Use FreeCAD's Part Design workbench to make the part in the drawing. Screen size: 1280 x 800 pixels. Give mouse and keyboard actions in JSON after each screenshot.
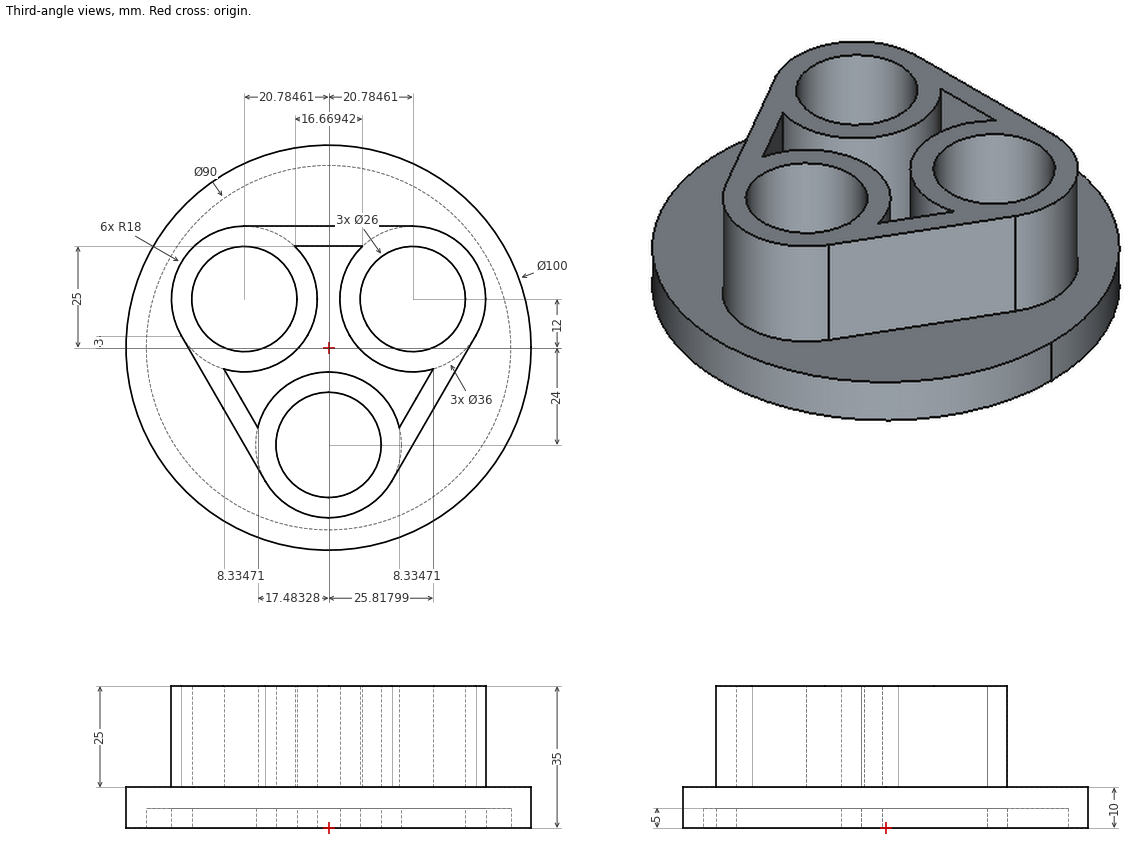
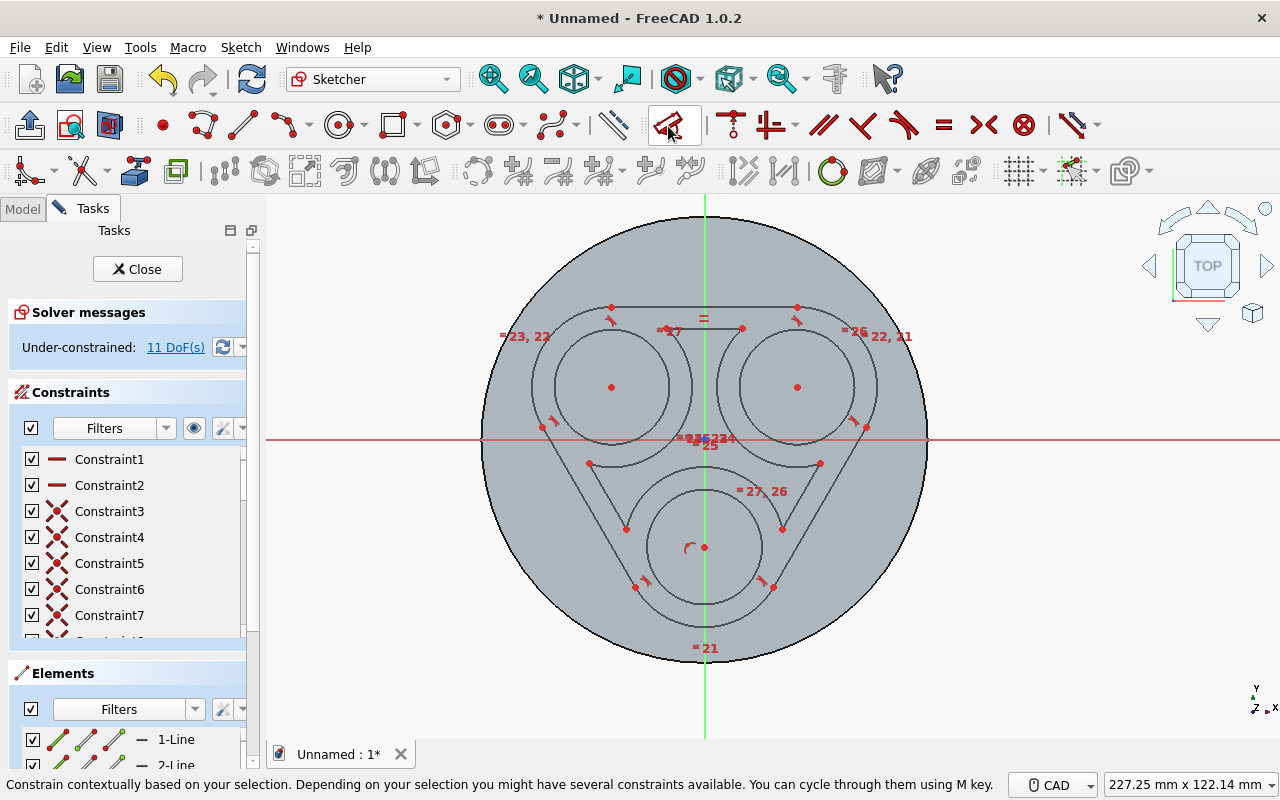
{"action": "left_click", "coordinate": [672, 620]}
{"action": "left_click", "coordinate": [659, 649]}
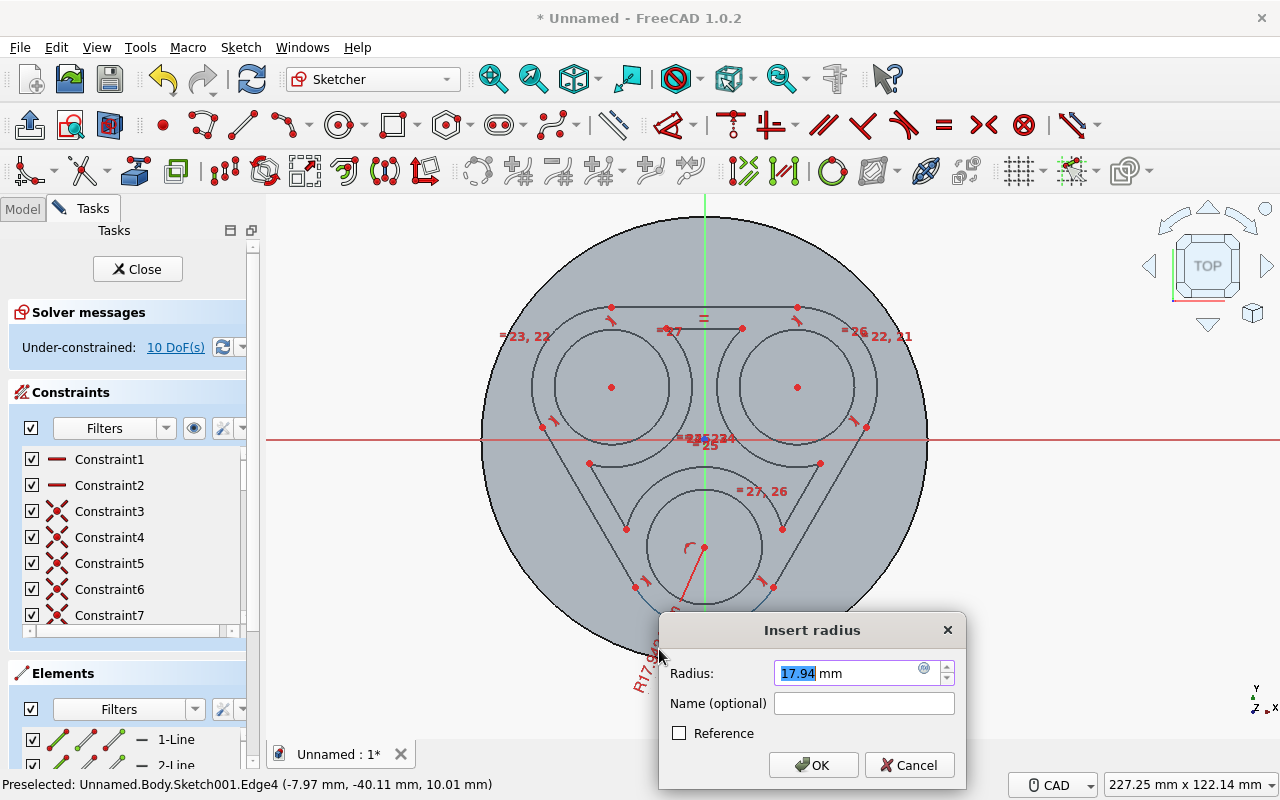
{"action": "type", "text": "18"}
{"action": "key", "text": "Return"}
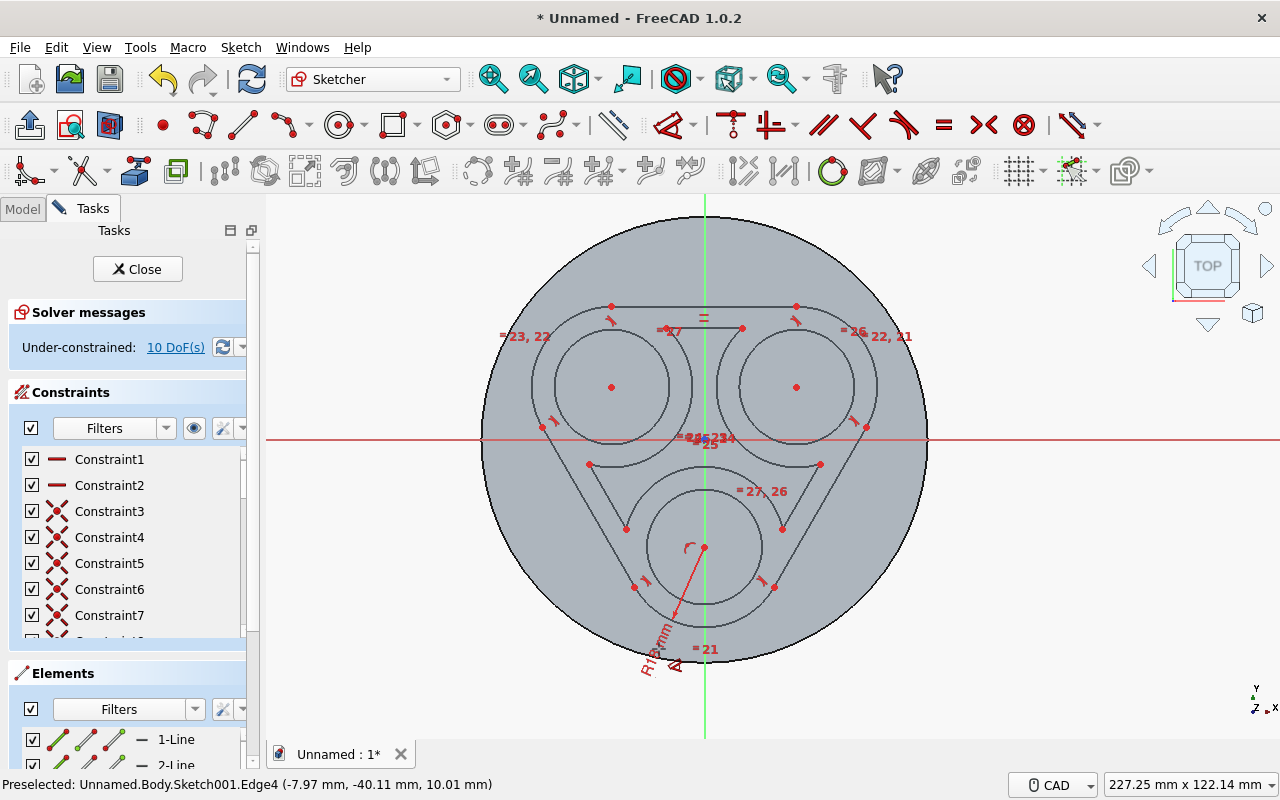
{"action": "left_click", "coordinate": [837, 346]}
{"action": "left_click", "coordinate": [875, 307]}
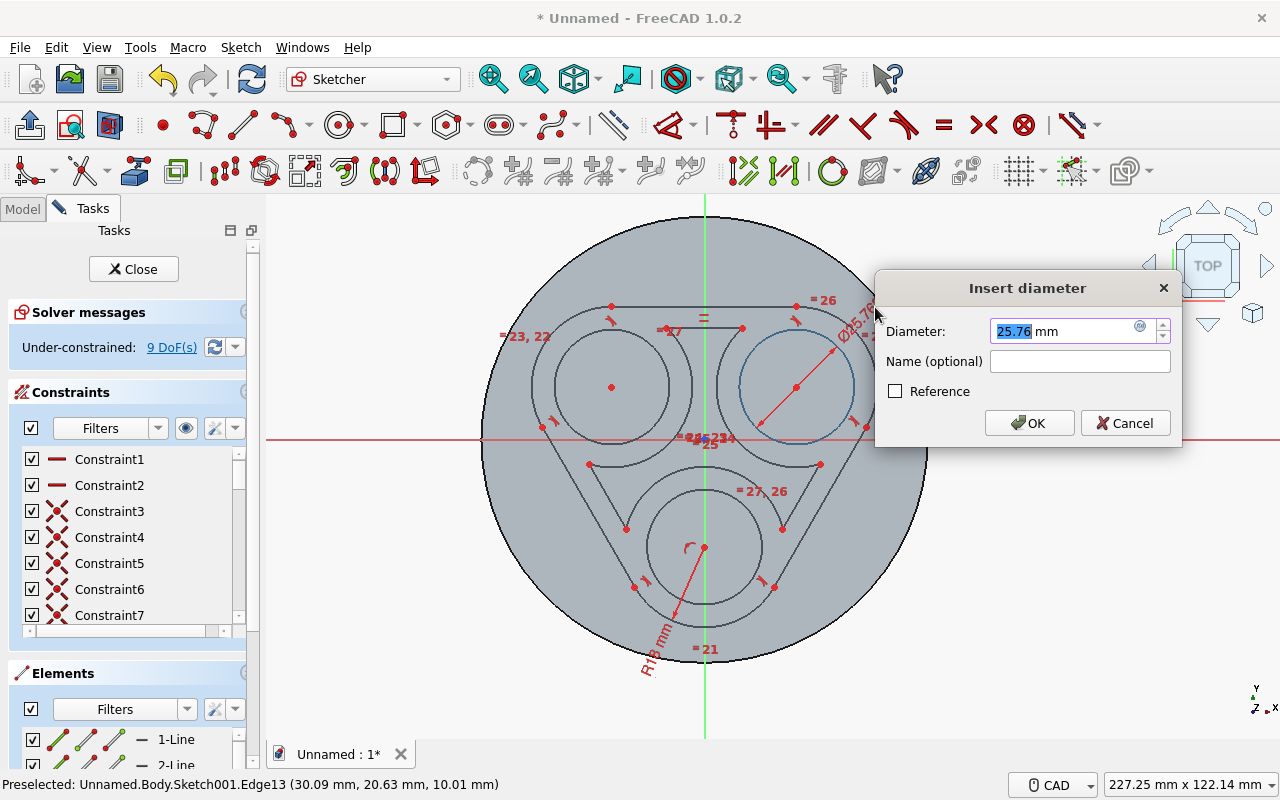
{"action": "type", "text": "26"}
{"action": "key", "text": "Return"}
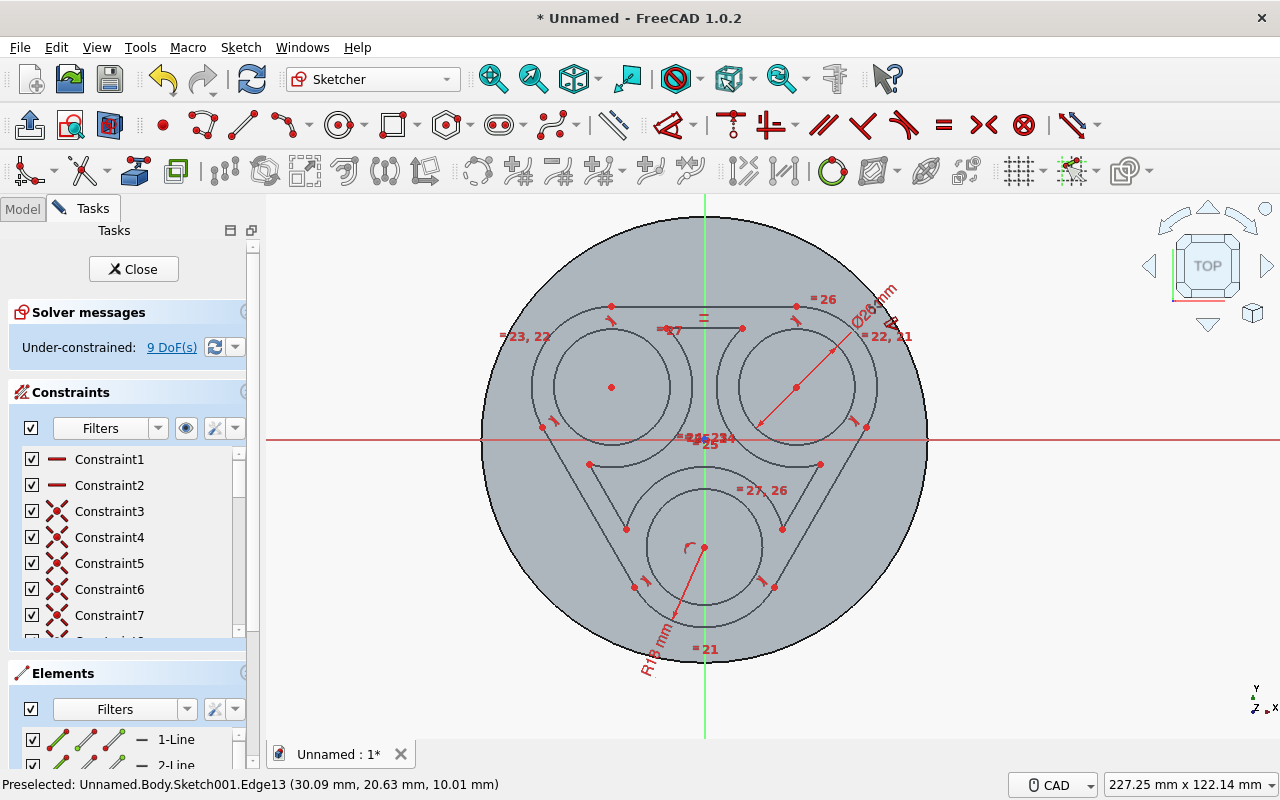
{"action": "scroll", "coordinate": [542, 427], "scroll_direction": "up", "scroll_amount": 6}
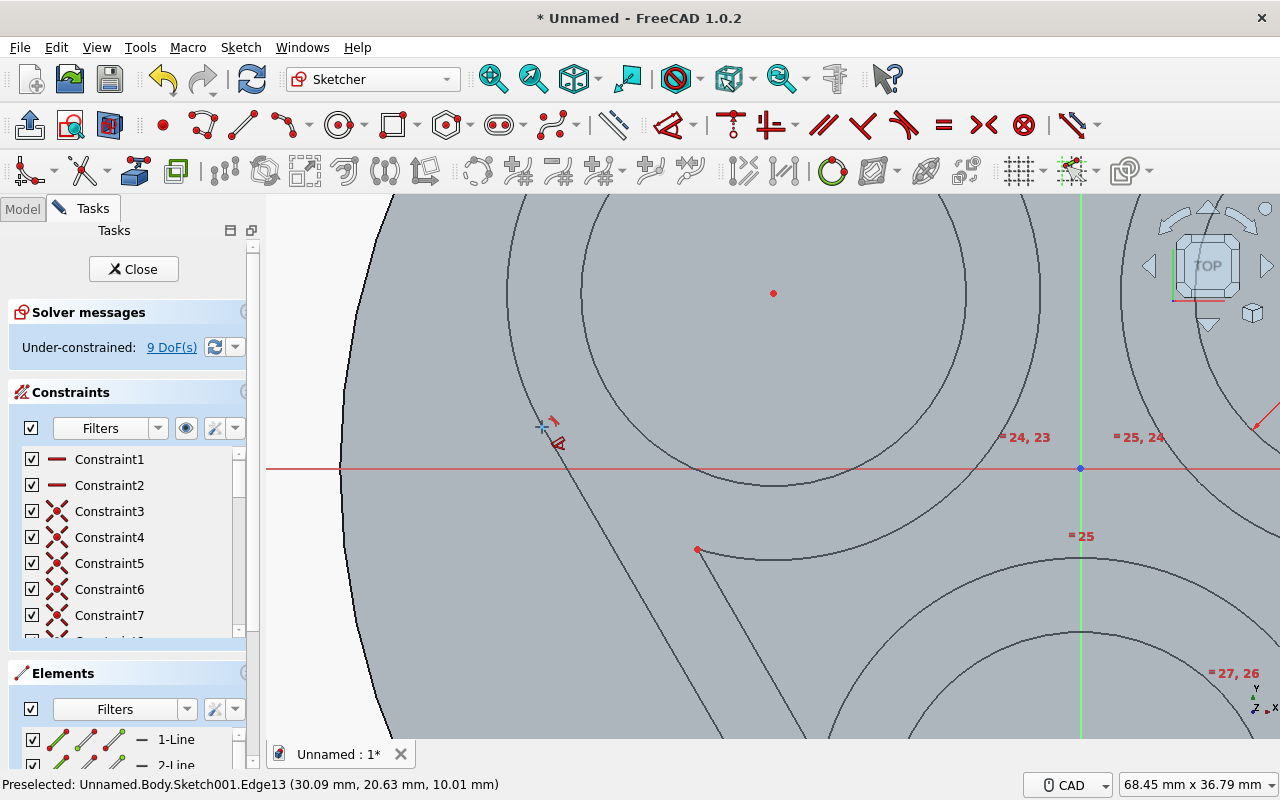
{"action": "left_click", "coordinate": [543, 427]}
{"action": "left_click", "coordinate": [509, 448]}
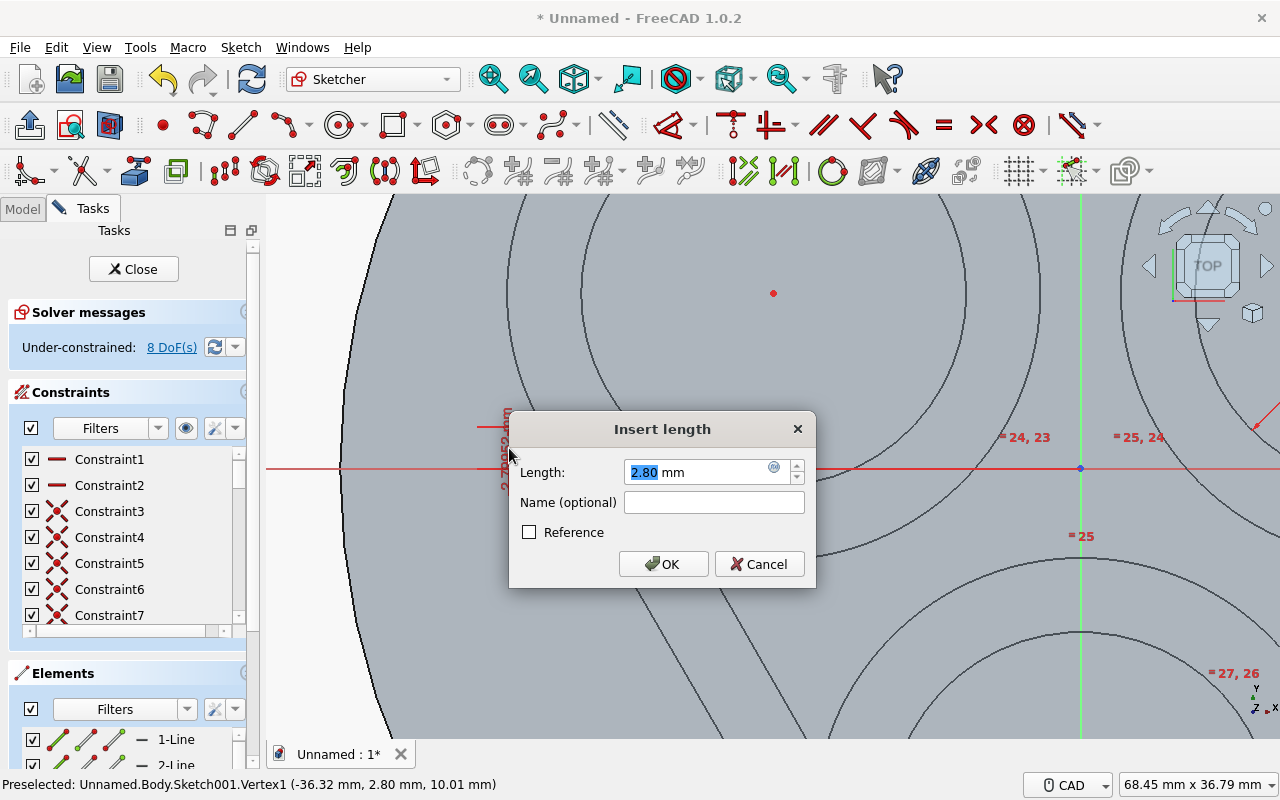
{"action": "type", "text": "3"}
{"action": "key", "text": "Return"}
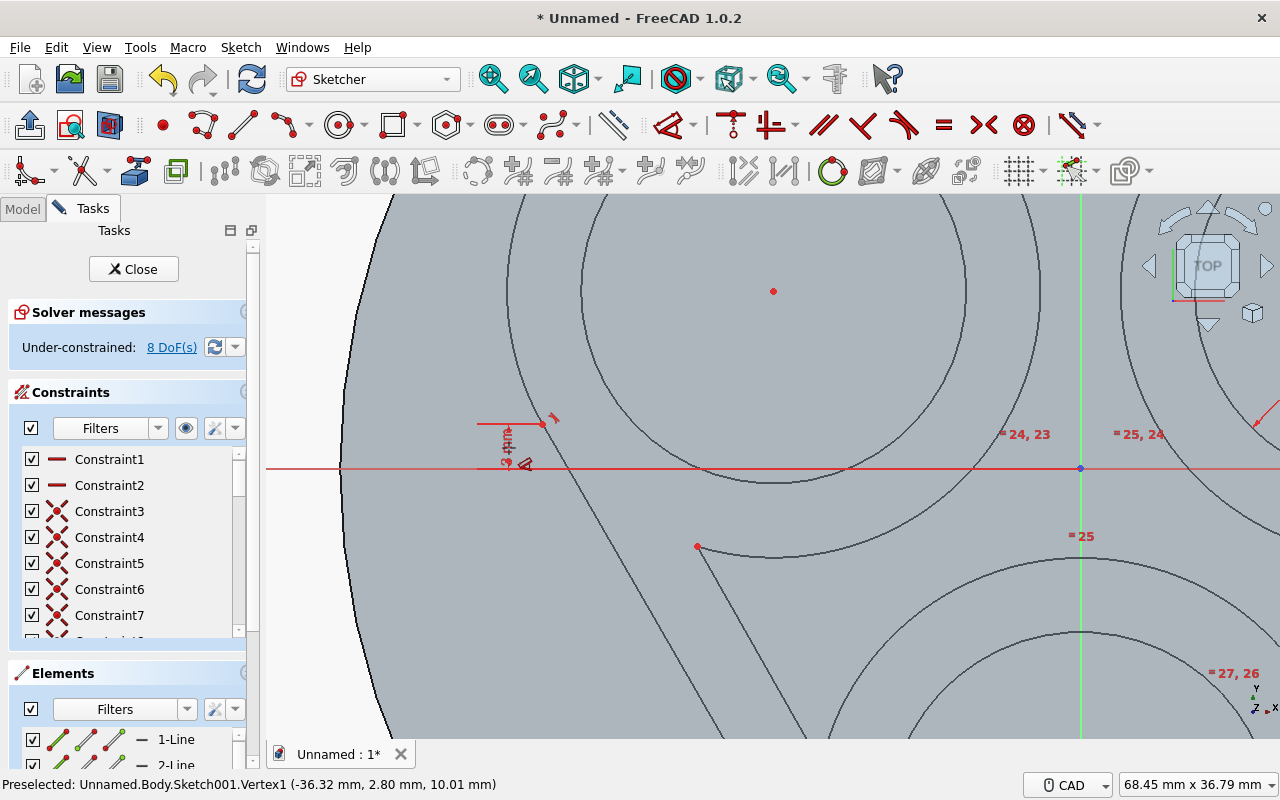
{"action": "scroll", "coordinate": [542, 427], "scroll_direction": "down", "scroll_amount": 6}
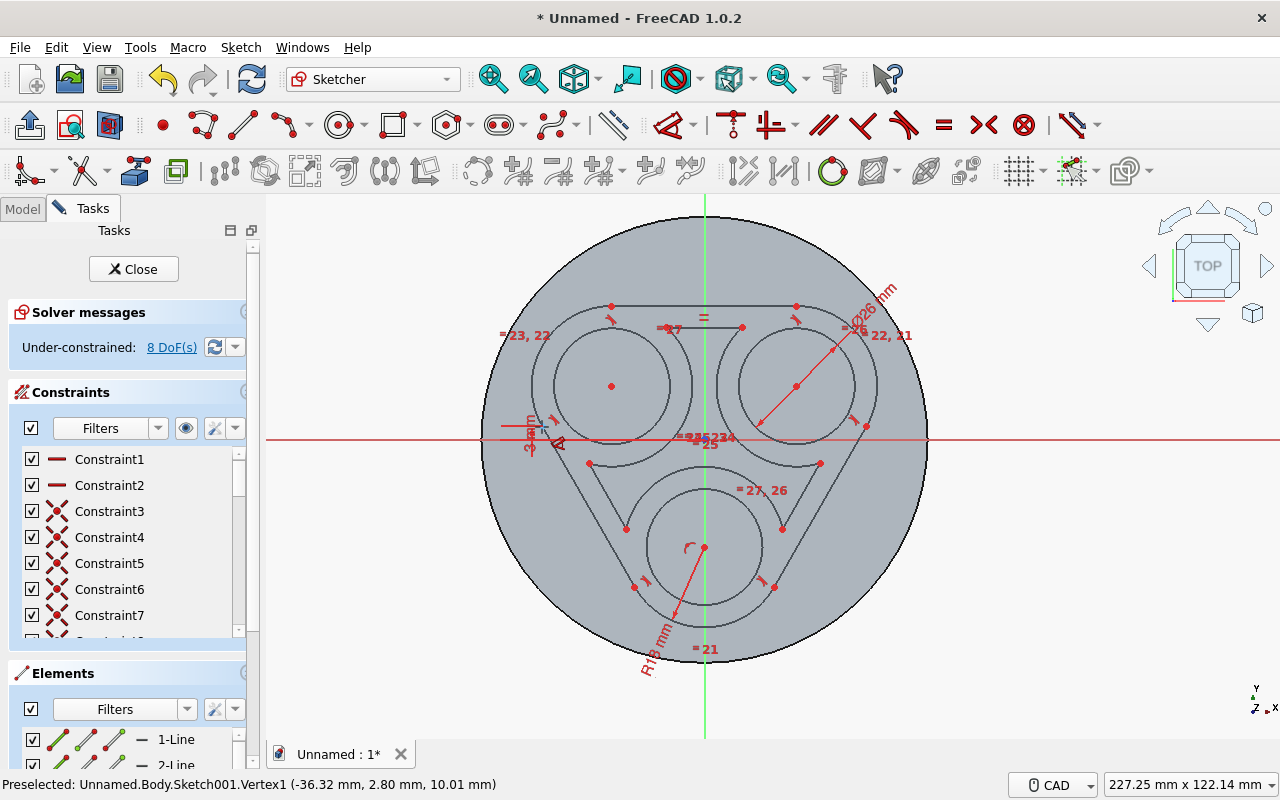
{"action": "scroll", "coordinate": [866, 426], "scroll_direction": "up", "scroll_amount": 6}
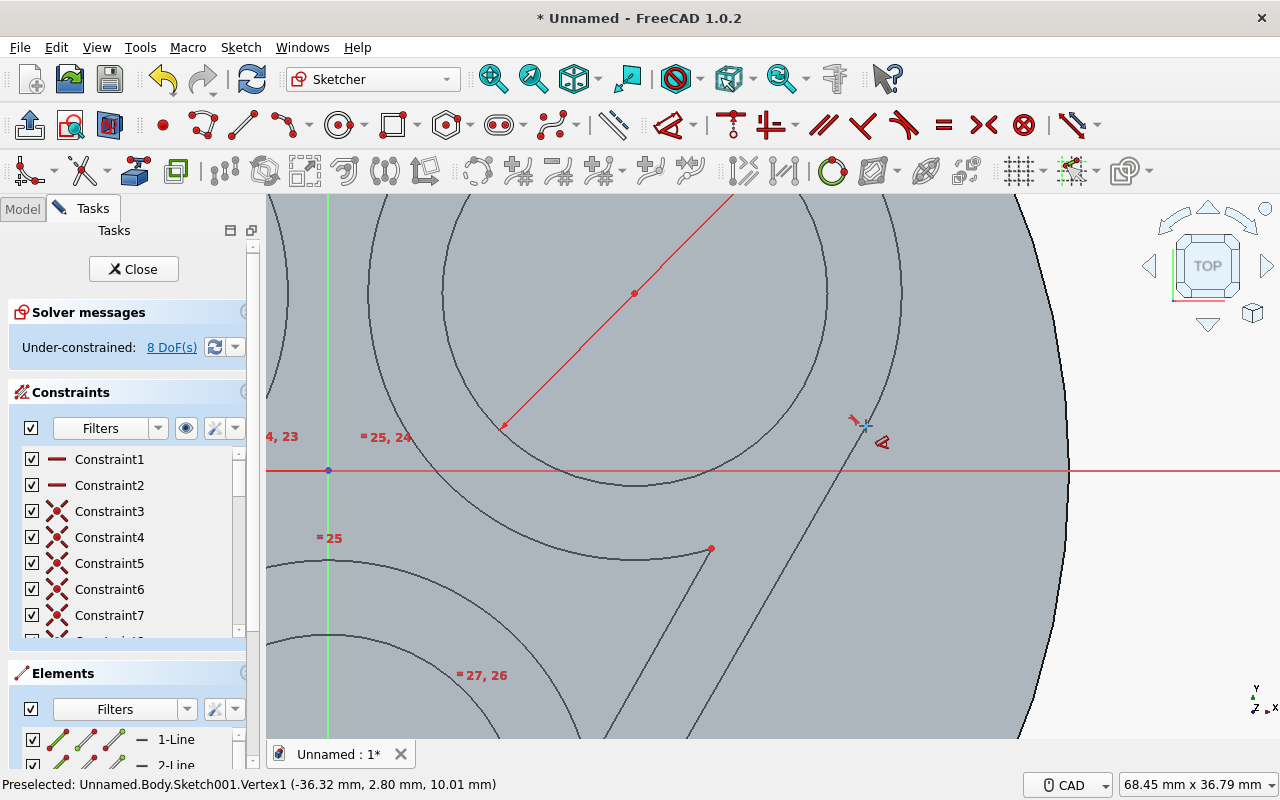
{"action": "left_click", "coordinate": [866, 426]}
{"action": "left_click", "coordinate": [900, 449]}